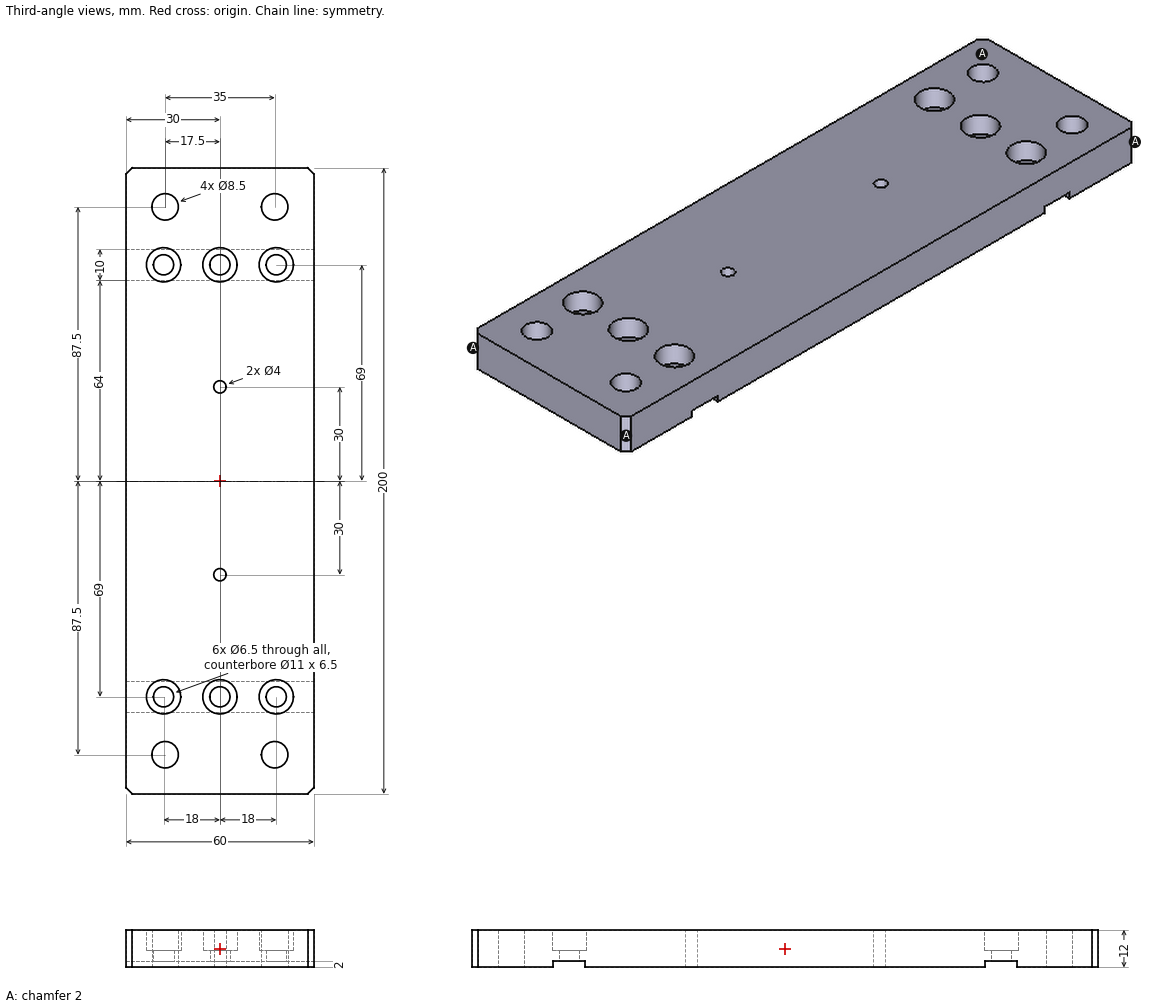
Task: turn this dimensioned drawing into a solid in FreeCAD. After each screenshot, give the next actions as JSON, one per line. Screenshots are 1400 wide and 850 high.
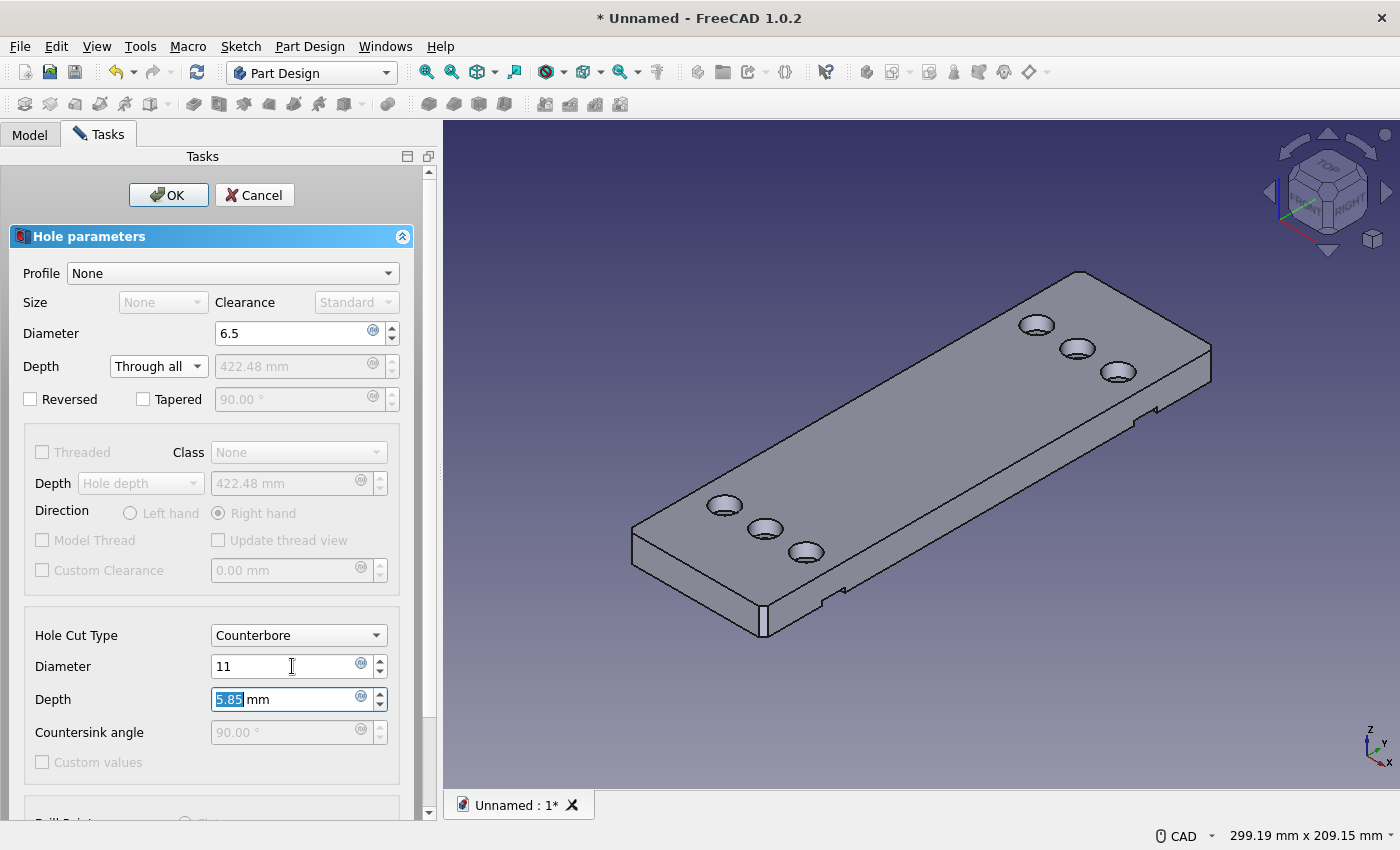
{"action": "type", "text": "6.5"}
{"action": "key", "text": "Tab"}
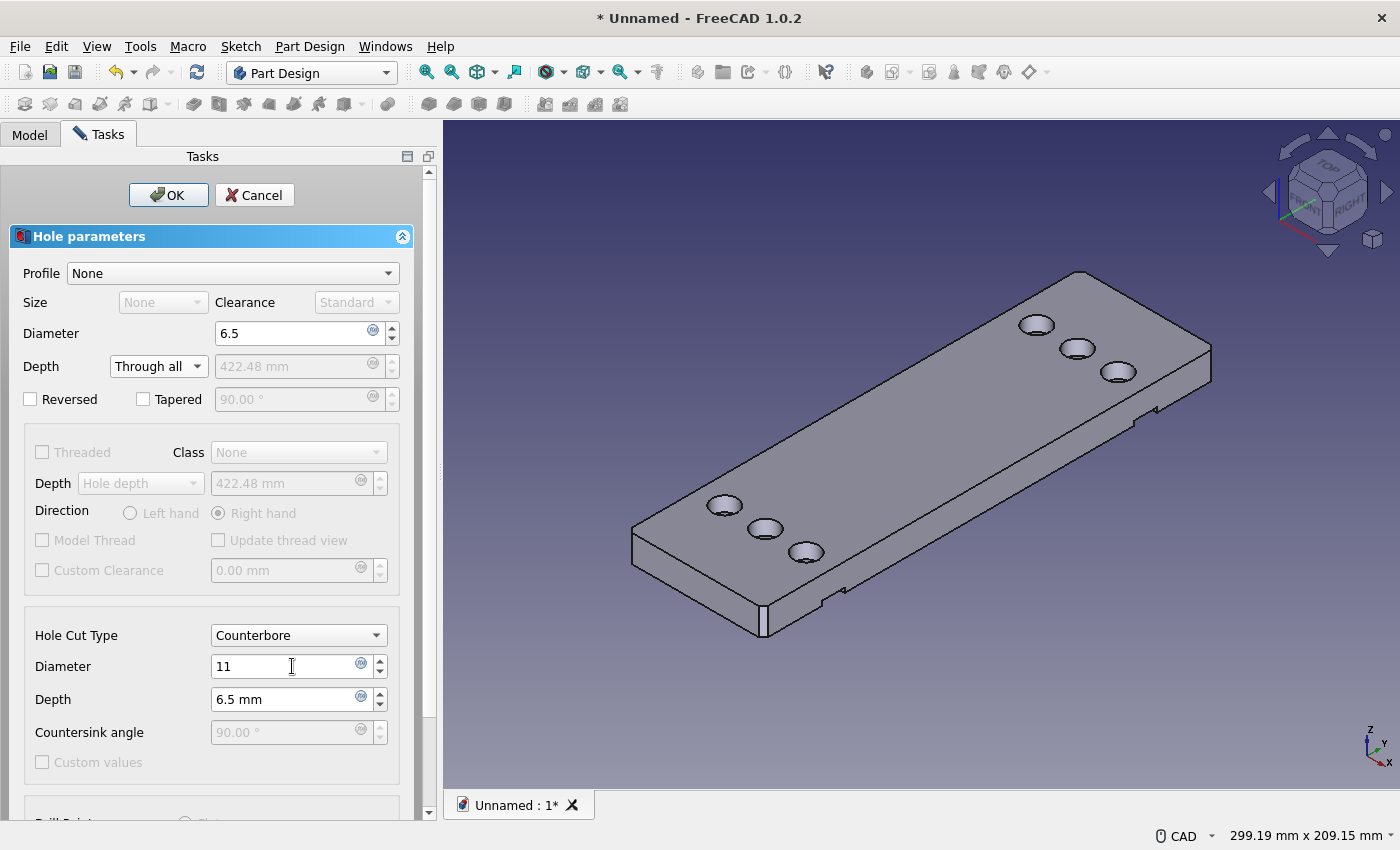
{"action": "left_click", "coordinate": [169, 195]}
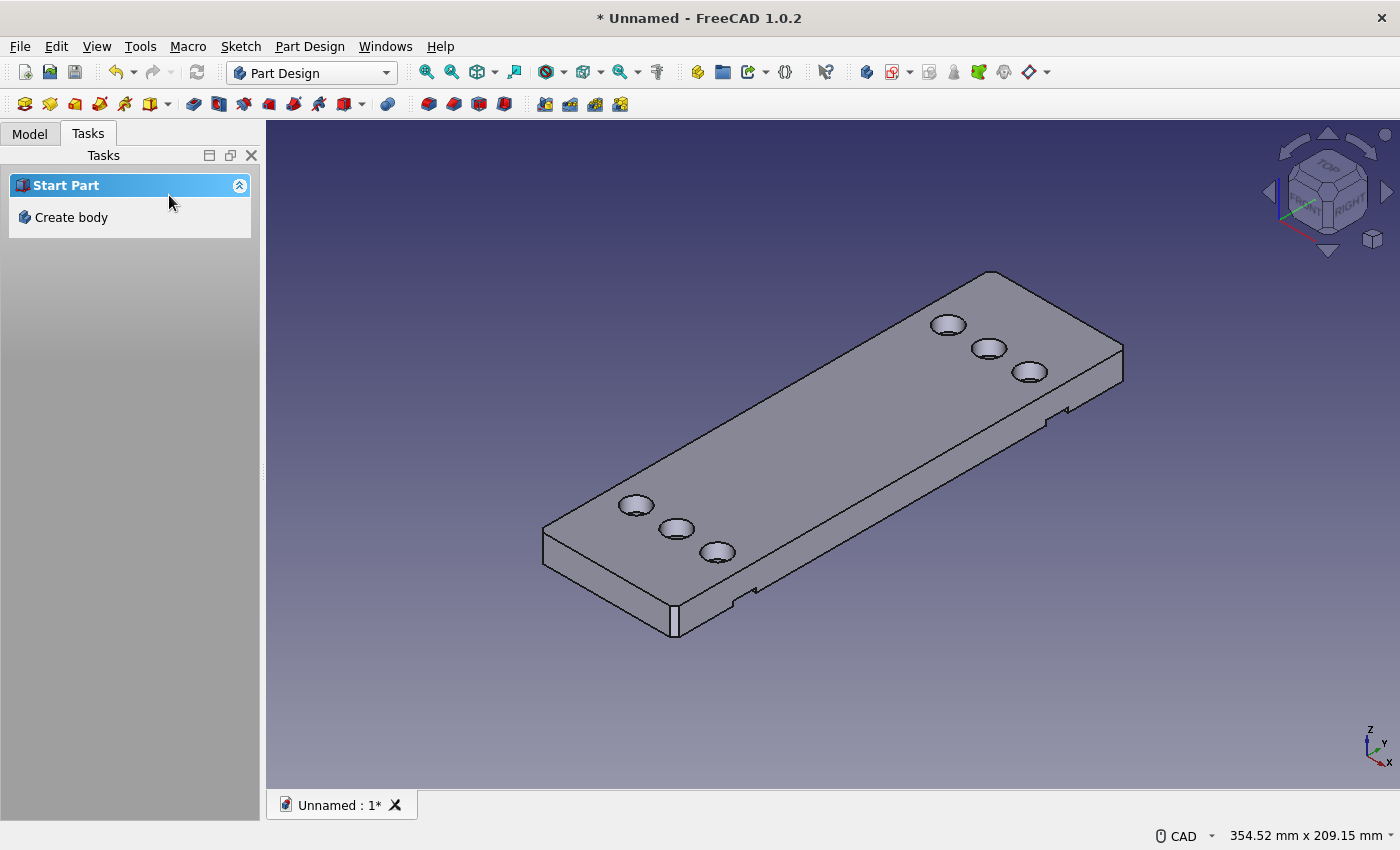
{"action": "key", "text": "5"}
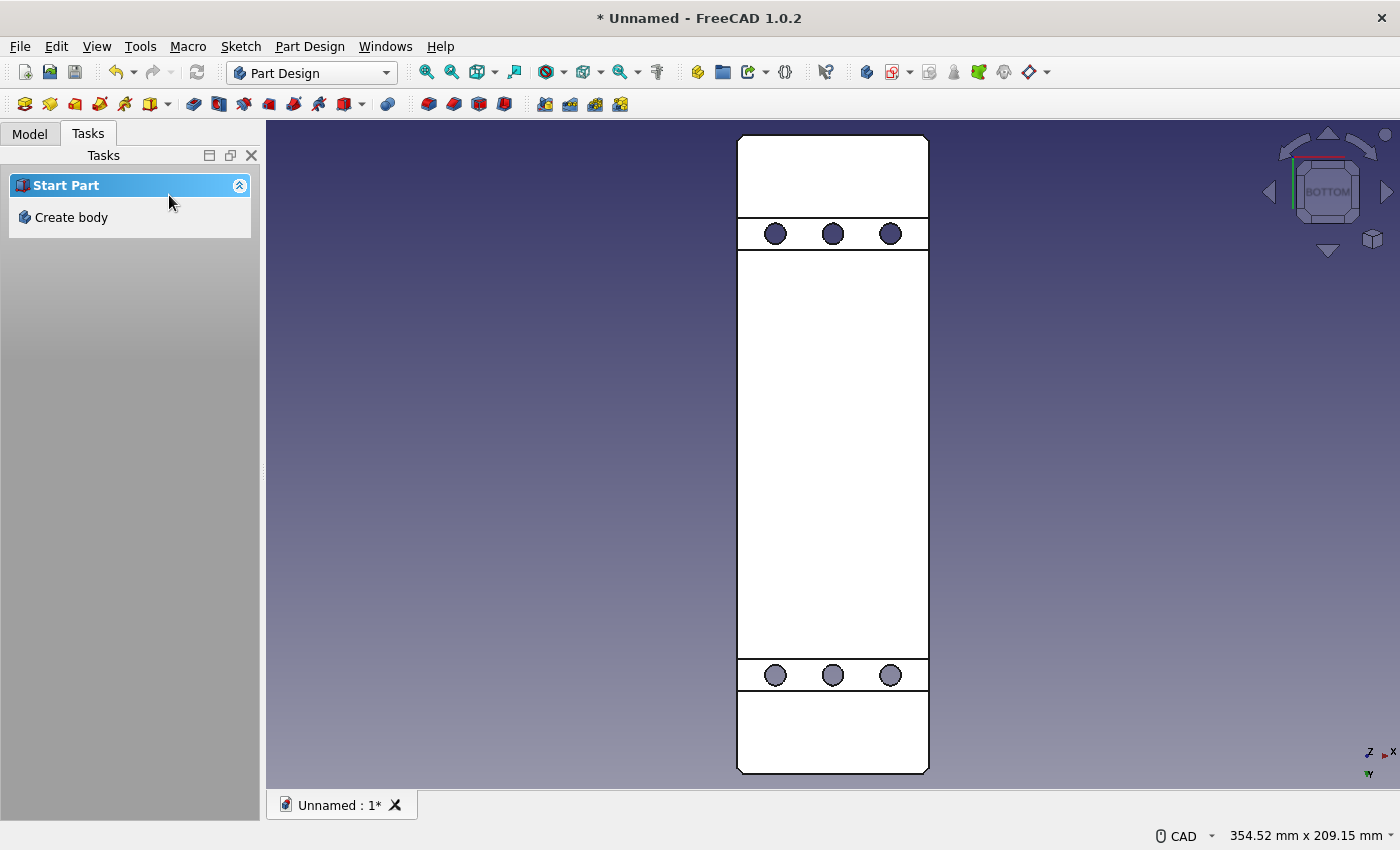
{"action": "left_click", "coordinate": [833, 512]}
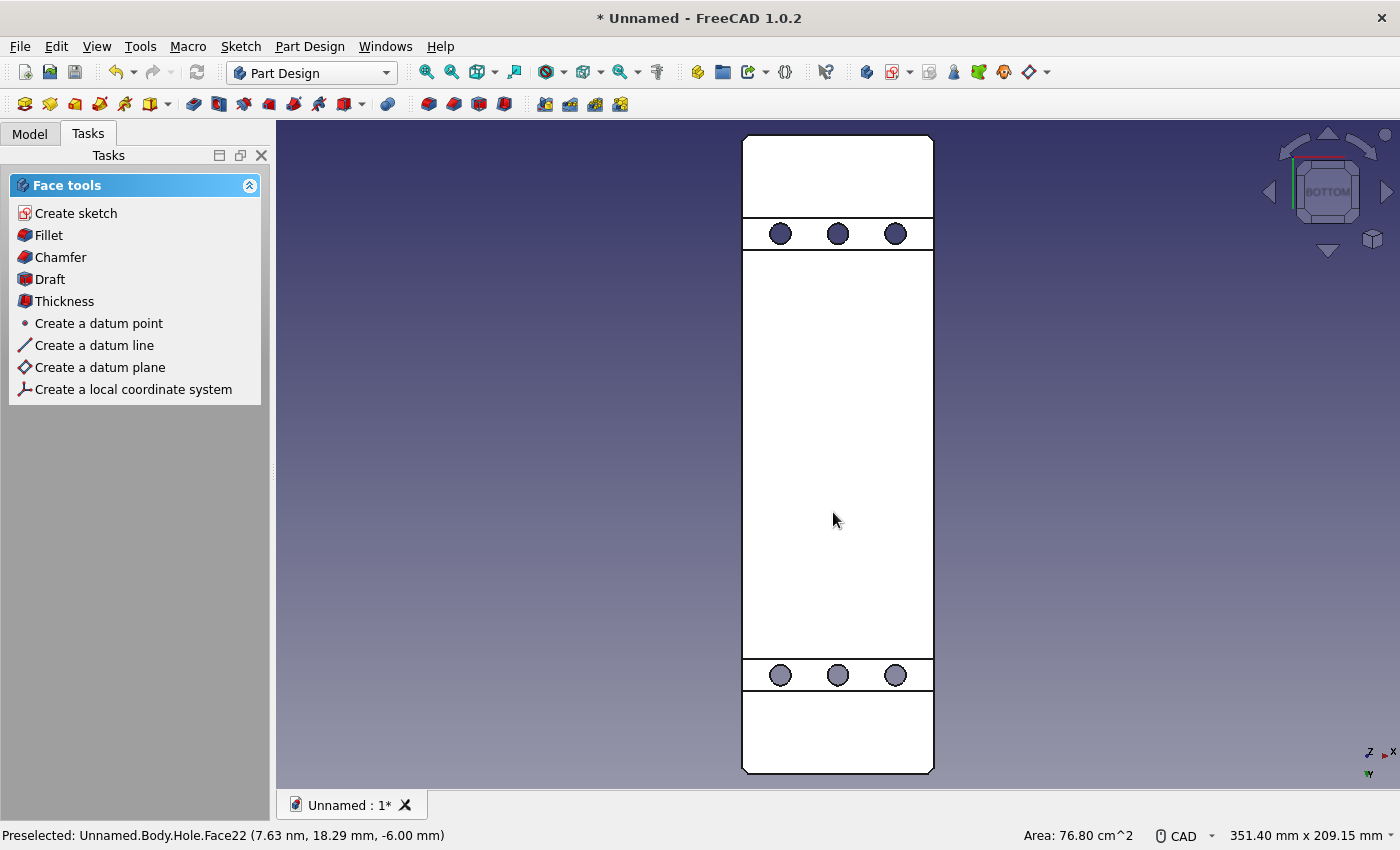
{"action": "left_click", "coordinate": [892, 72]}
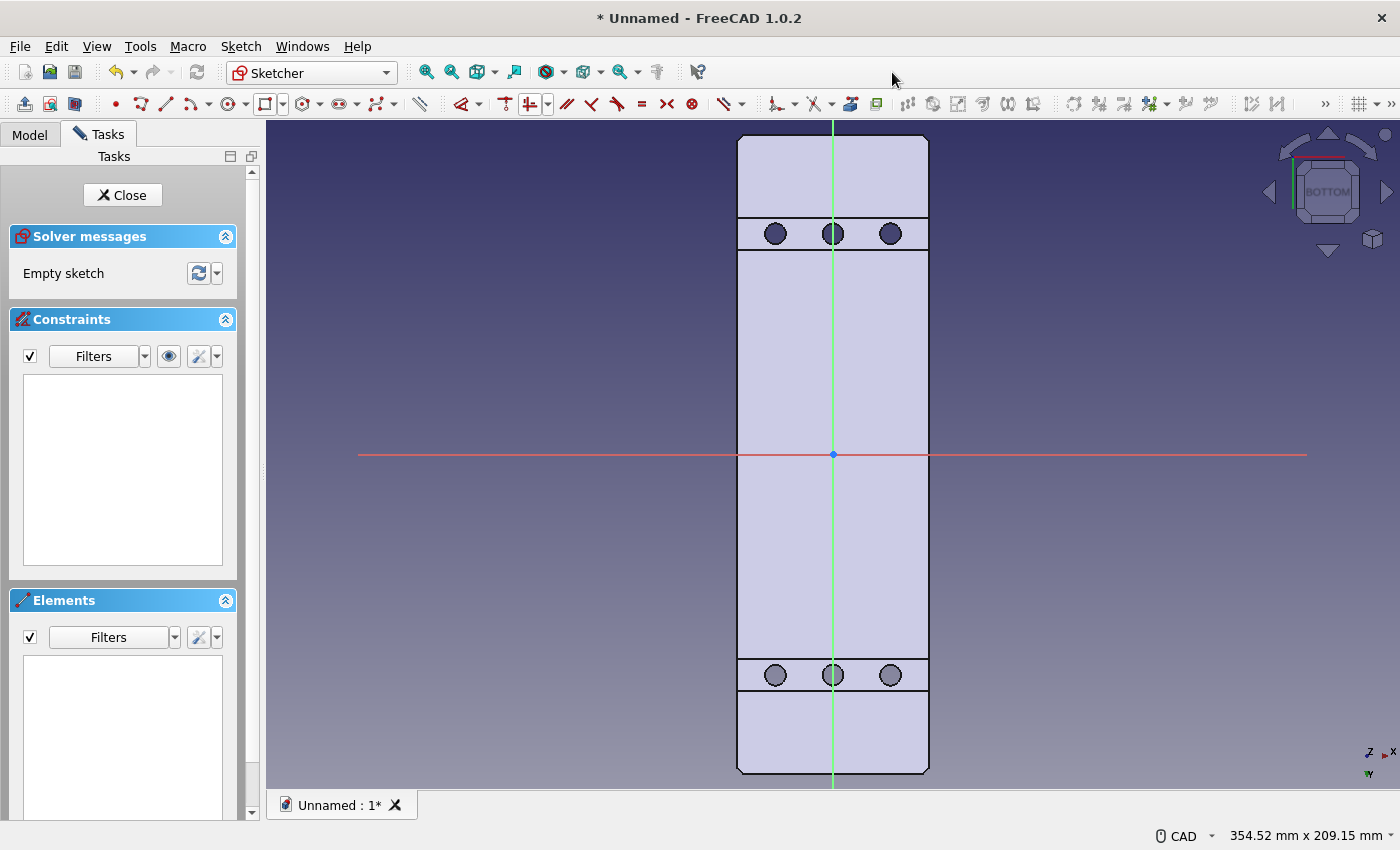
{"action": "scroll", "coordinate": [625, 454], "scroll_direction": "down", "scroll_amount": 2}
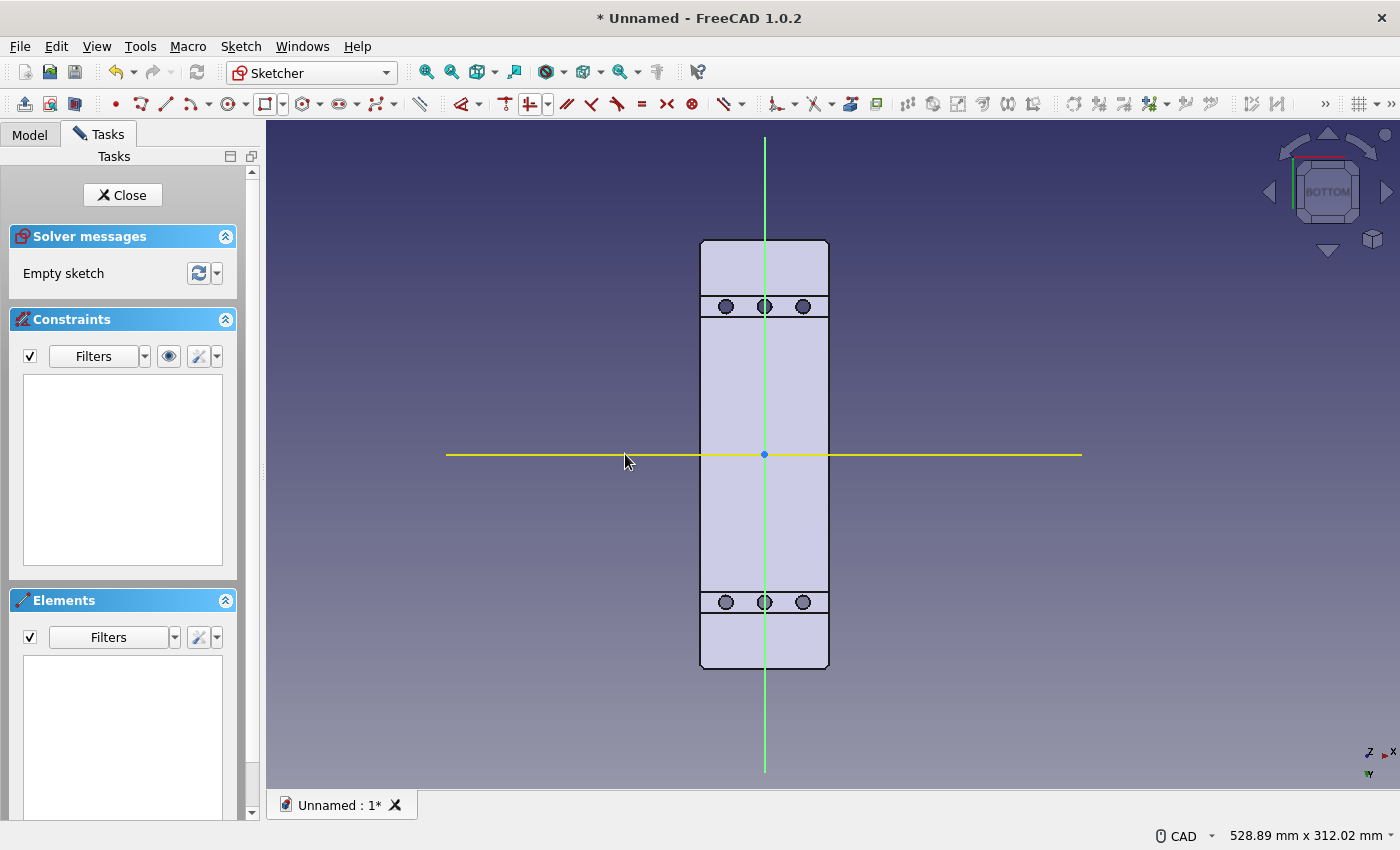
{"action": "left_click", "coordinate": [228, 104]}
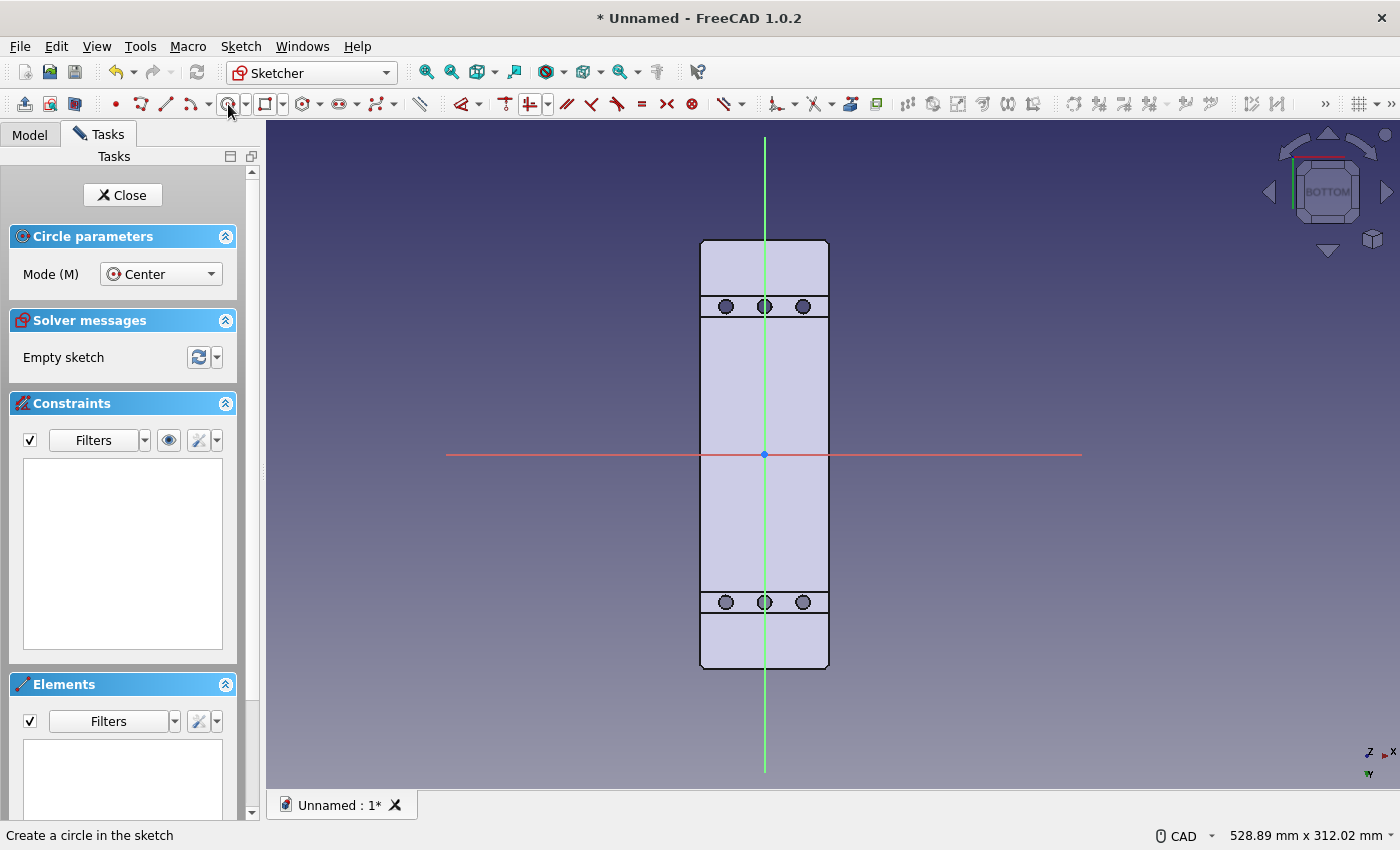
{"action": "scroll", "coordinate": [727, 642], "scroll_direction": "up", "scroll_amount": 5}